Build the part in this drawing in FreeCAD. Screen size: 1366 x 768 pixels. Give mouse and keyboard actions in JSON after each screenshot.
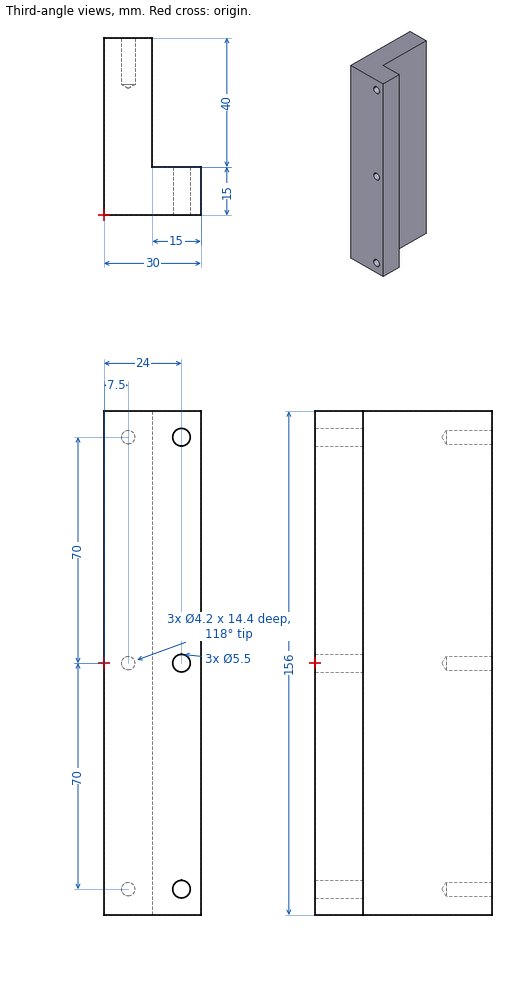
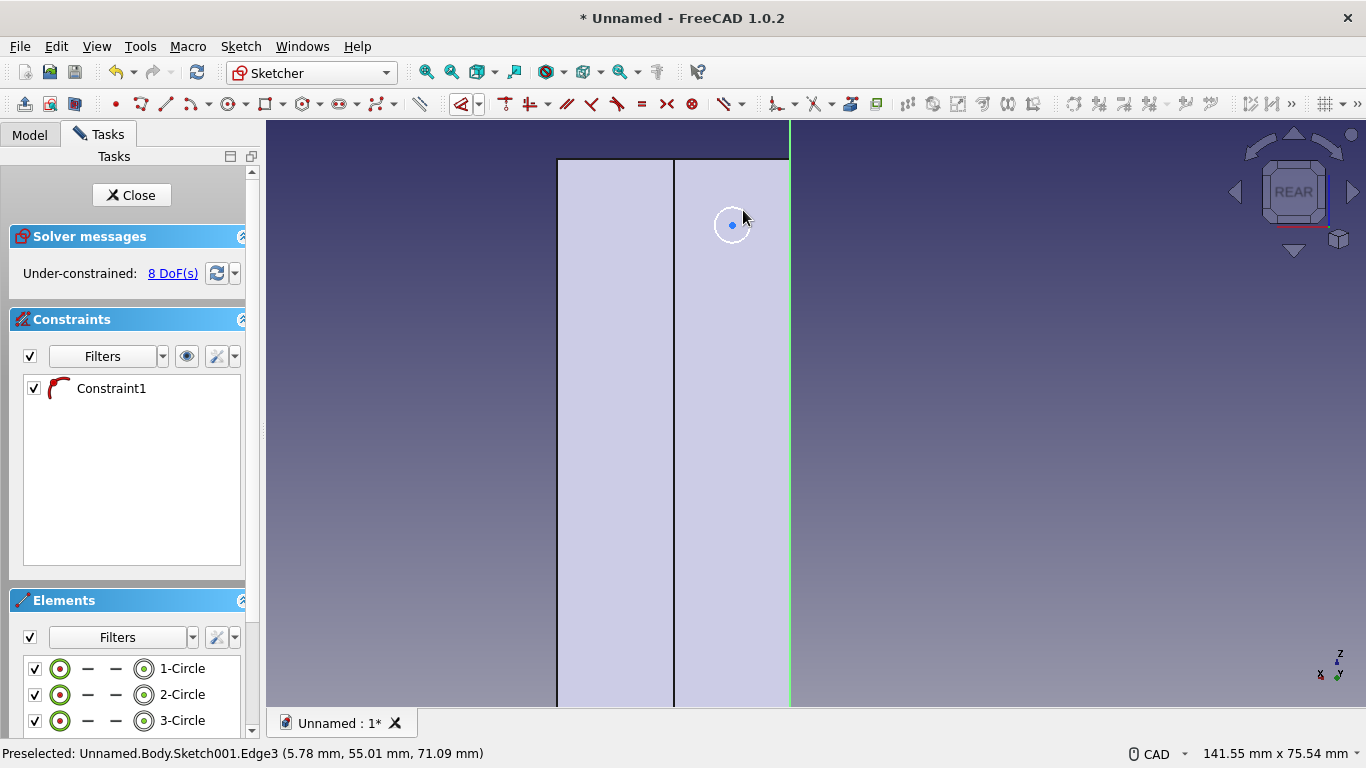
{"action": "scroll", "coordinate": [744, 209], "scroll_direction": "down", "scroll_amount": 5}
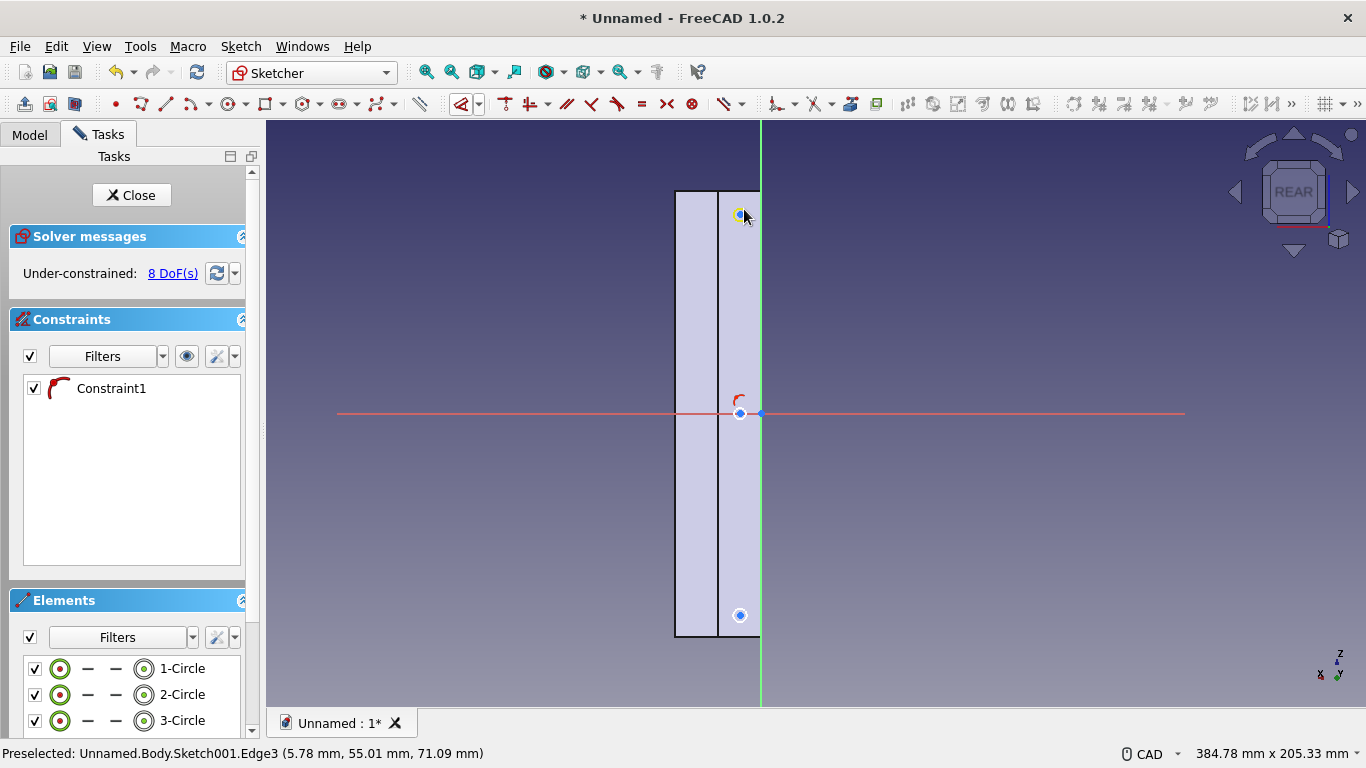
{"action": "scroll", "coordinate": [744, 410], "scroll_direction": "up", "scroll_amount": 7}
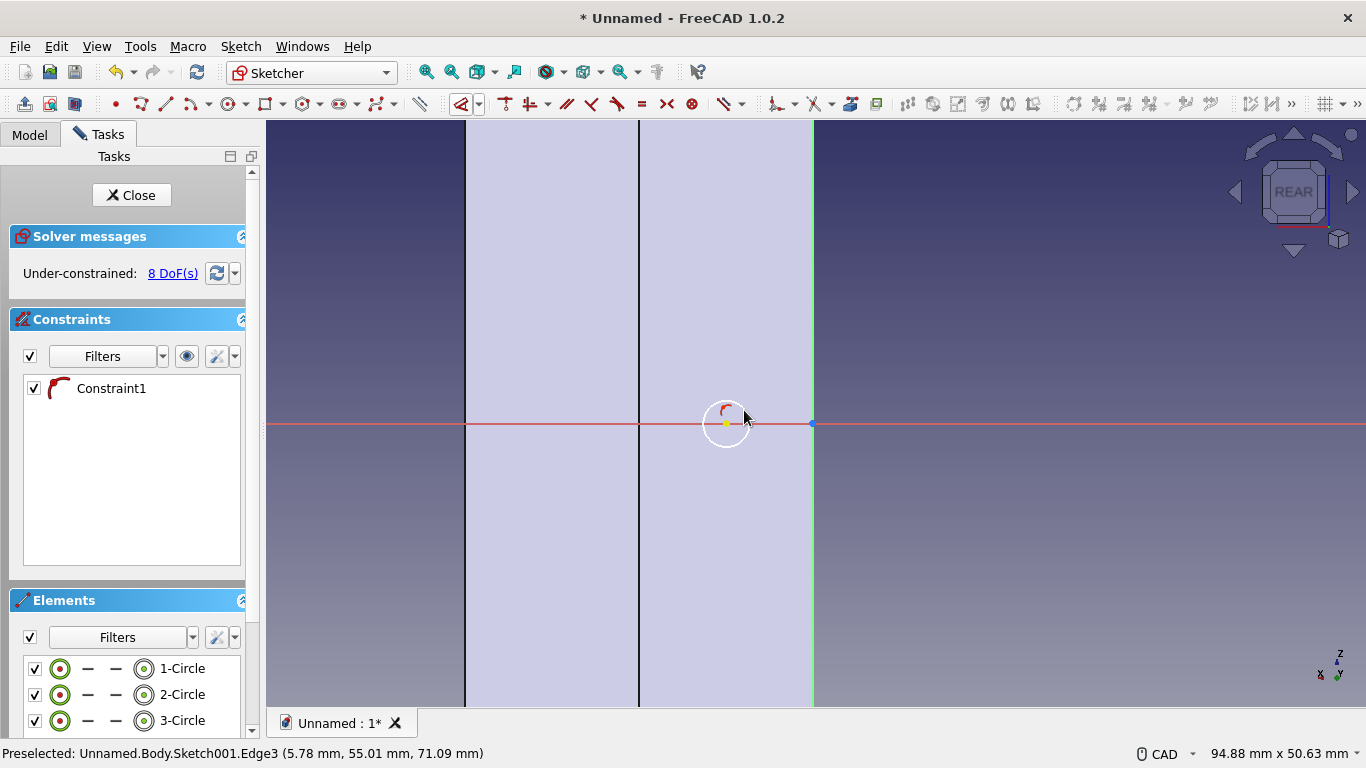
{"action": "left_click", "coordinate": [743, 408]}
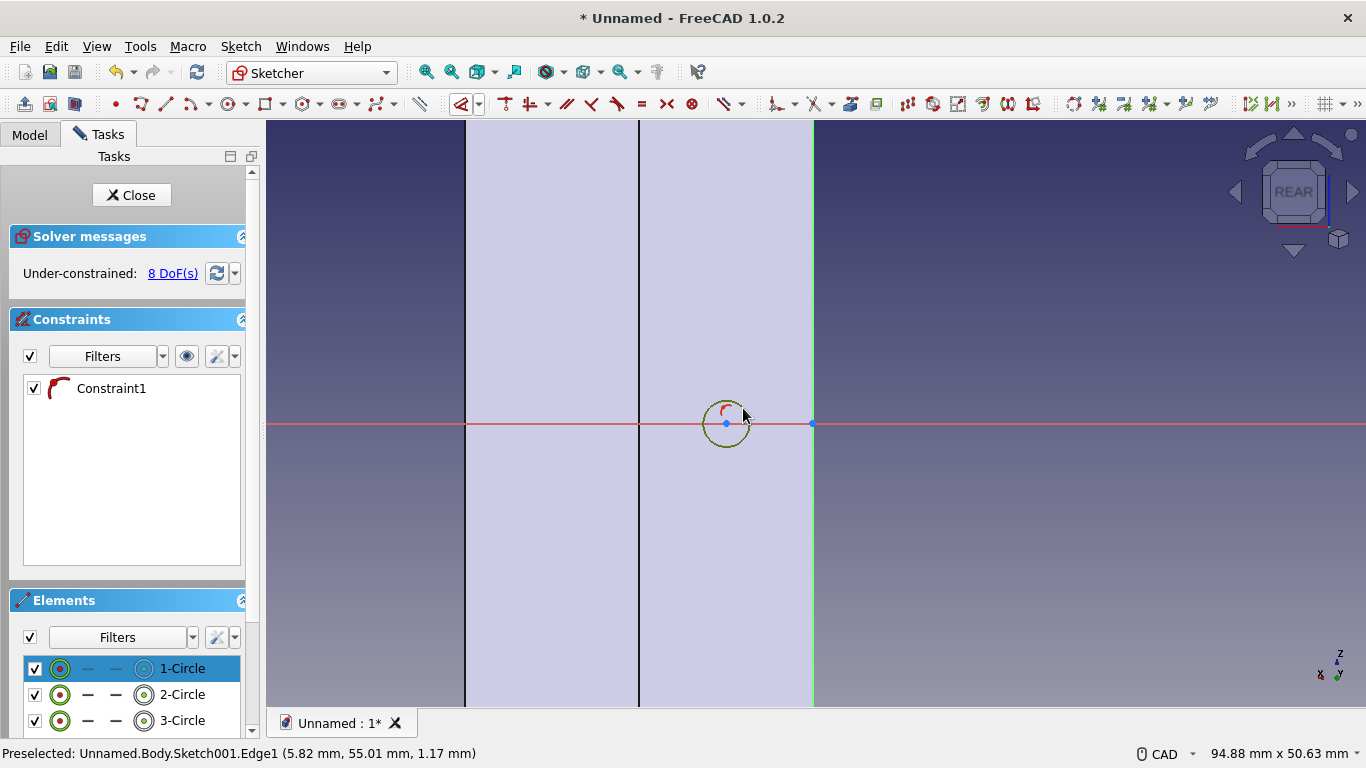
{"action": "scroll", "coordinate": [744, 410], "scroll_direction": "down", "scroll_amount": 7}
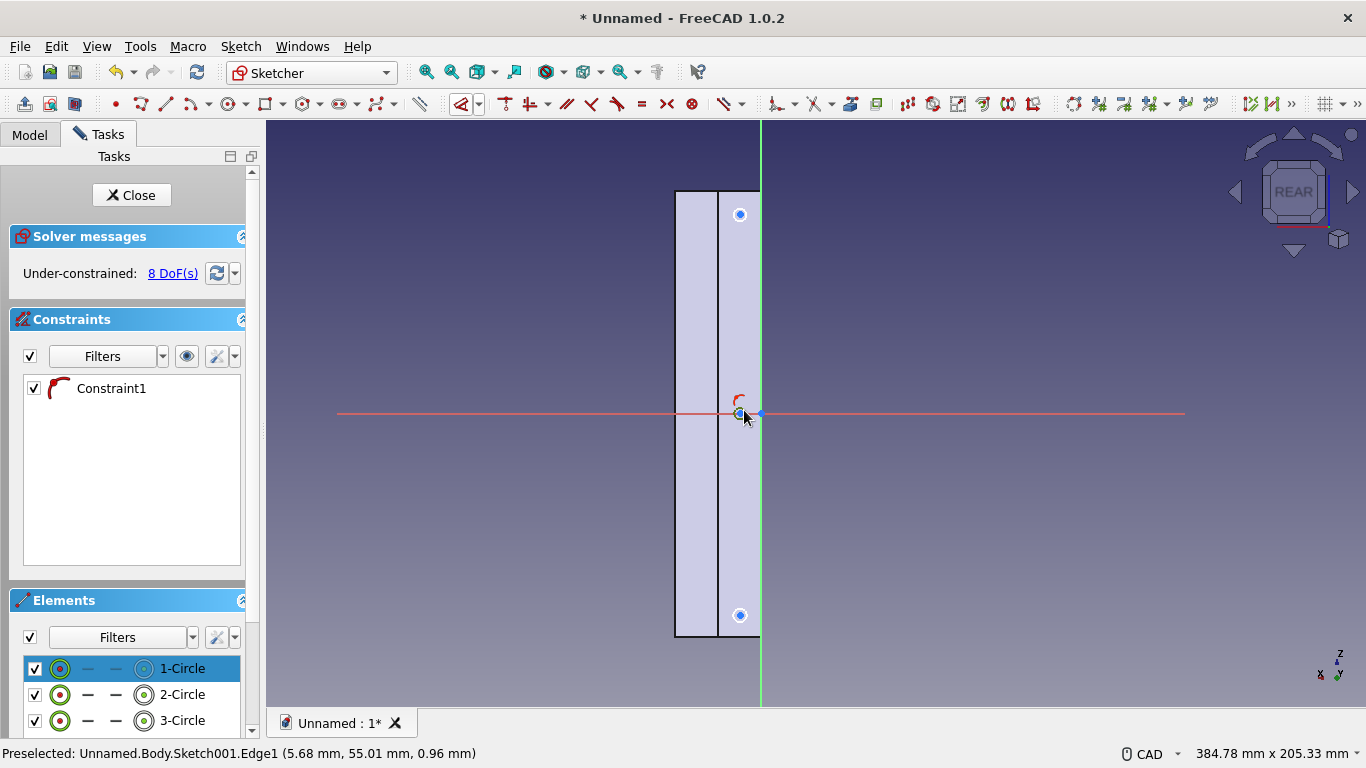
{"action": "scroll", "coordinate": [745, 611], "scroll_direction": "up", "scroll_amount": 4}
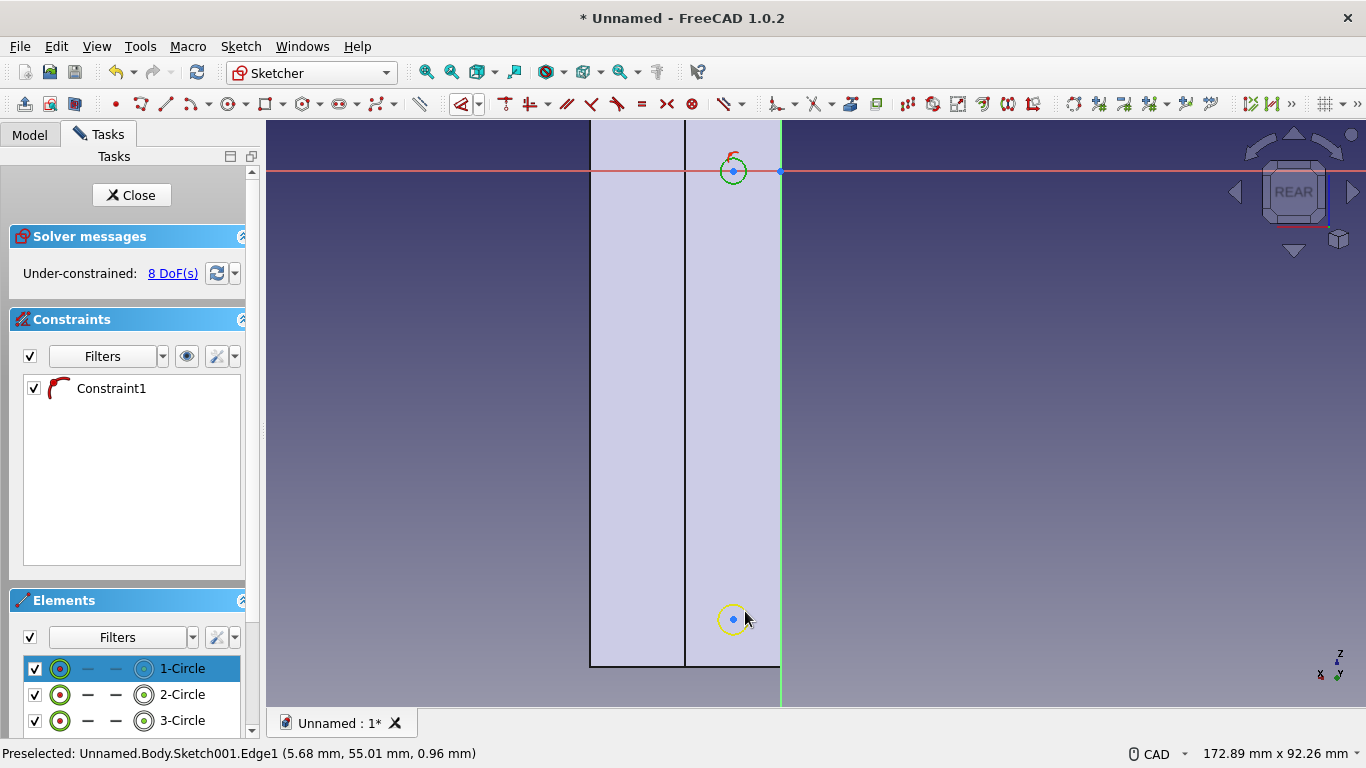
{"action": "left_click", "coordinate": [744, 609]}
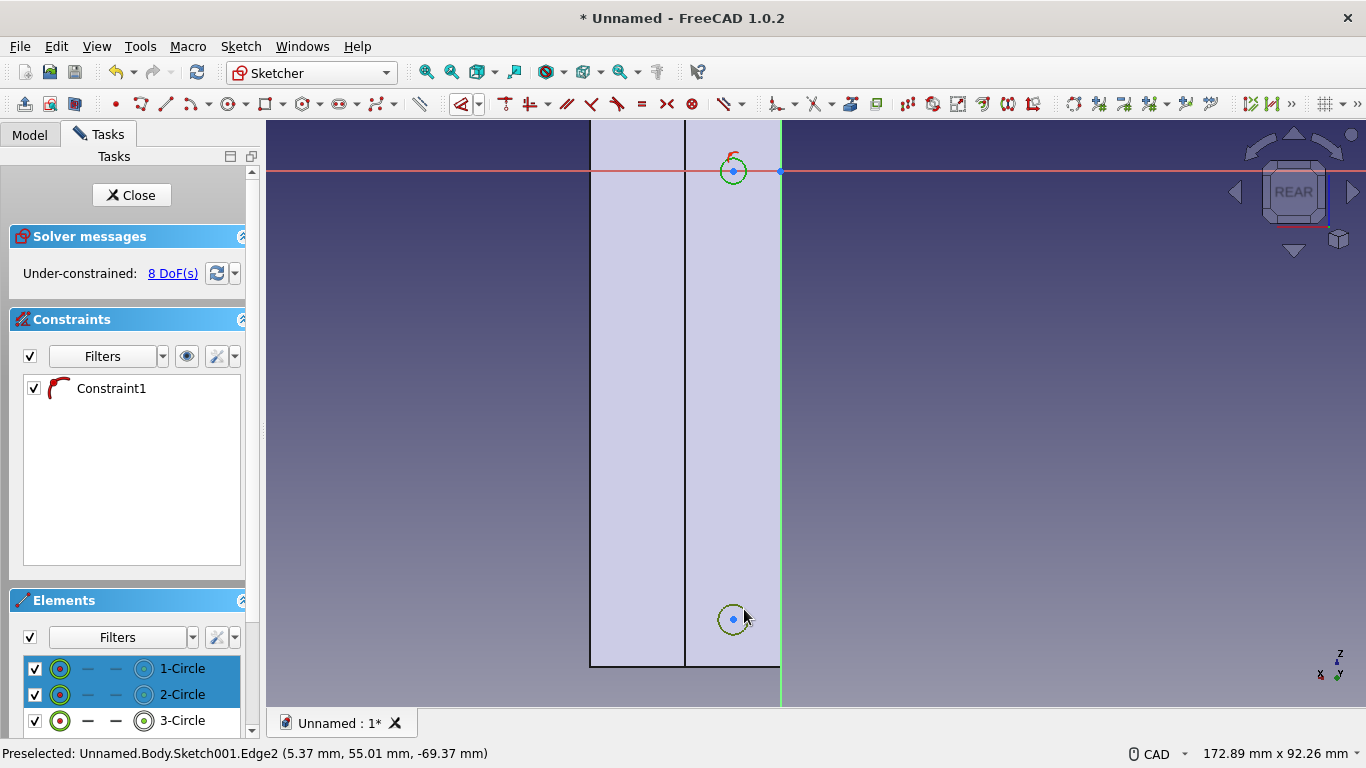
{"action": "scroll", "coordinate": [745, 611], "scroll_direction": "down", "scroll_amount": 4}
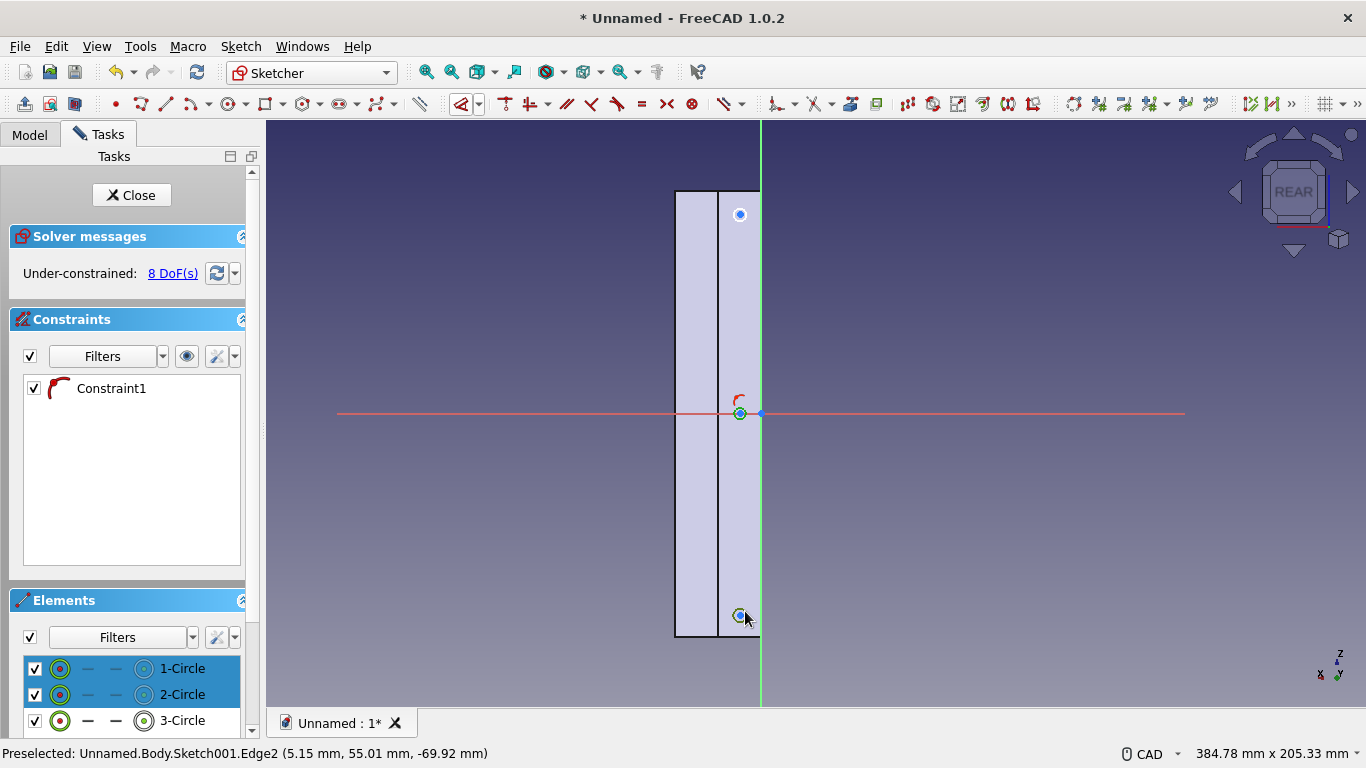
{"action": "scroll", "coordinate": [745, 210], "scroll_direction": "up", "scroll_amount": 4}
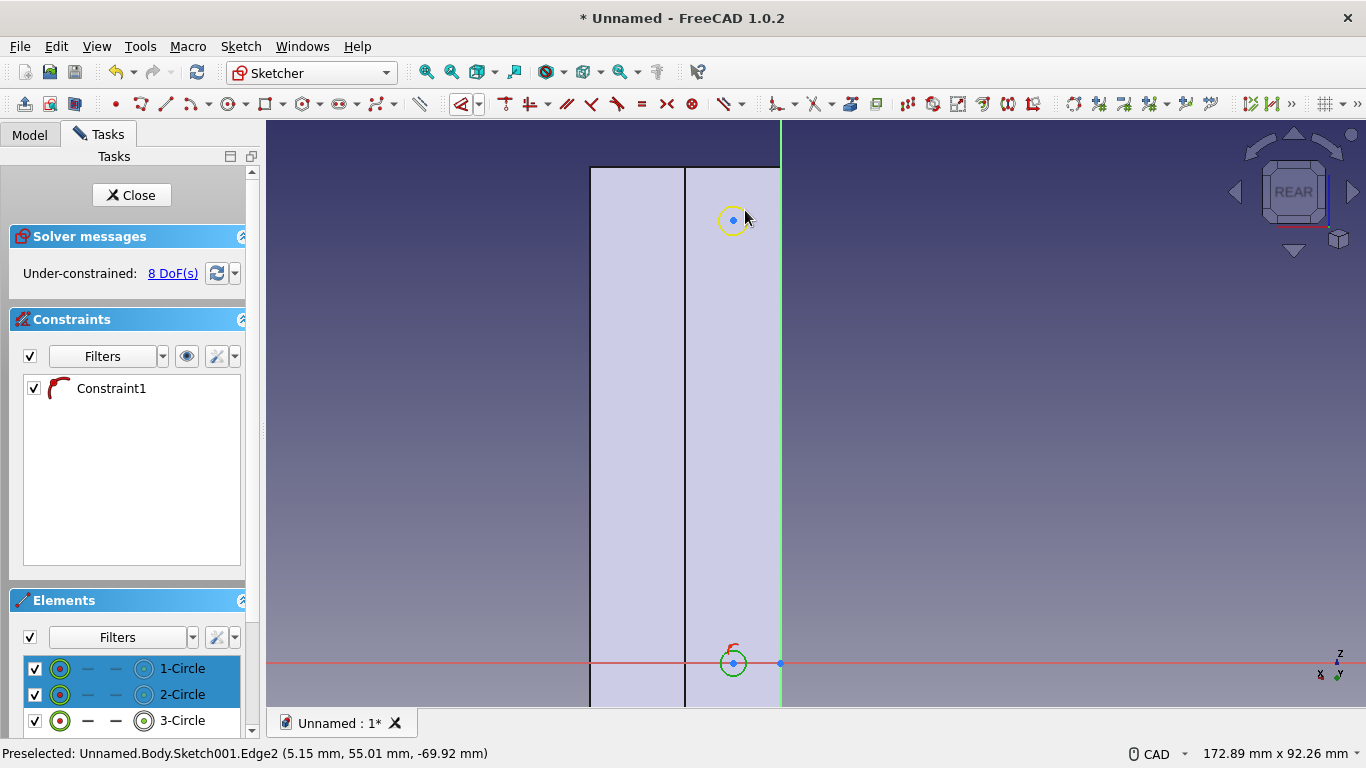
{"action": "left_click", "coordinate": [744, 211]}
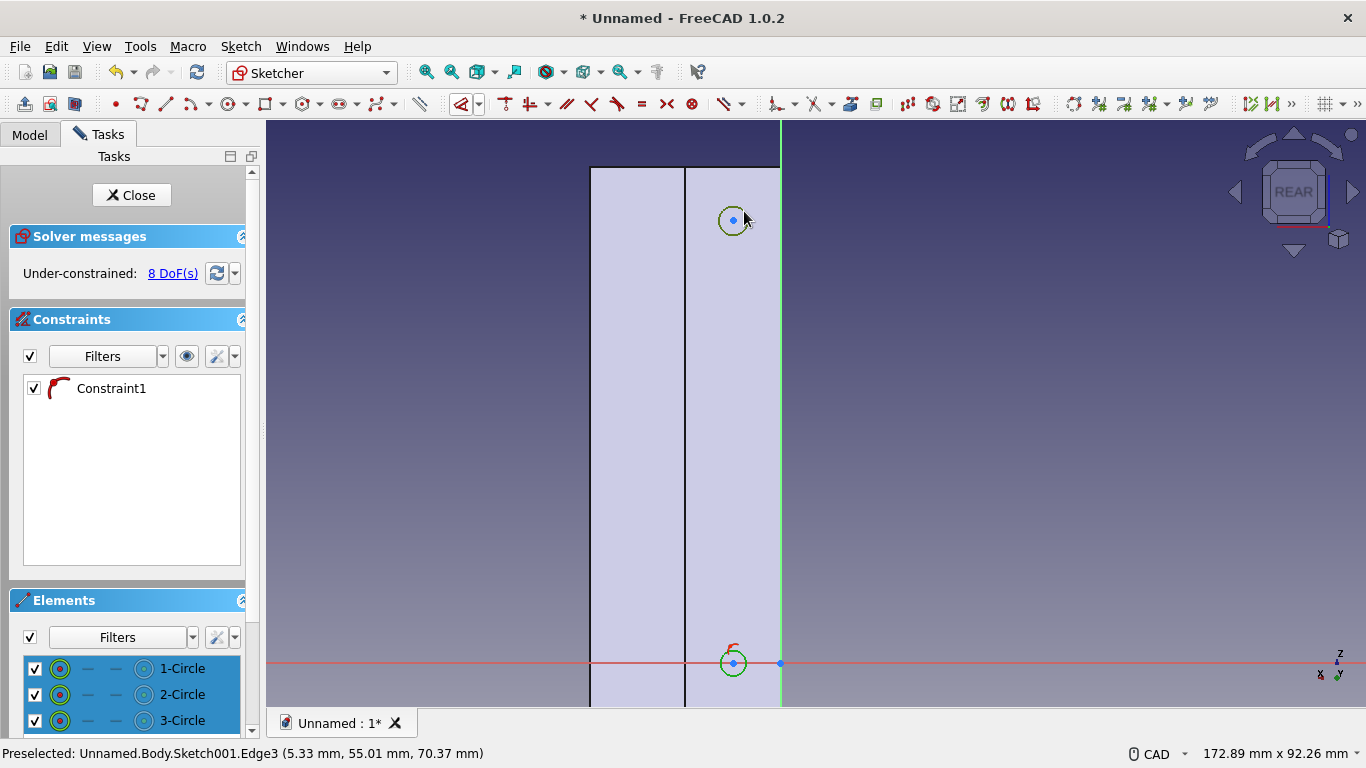
{"action": "left_click", "coordinate": [642, 104]}